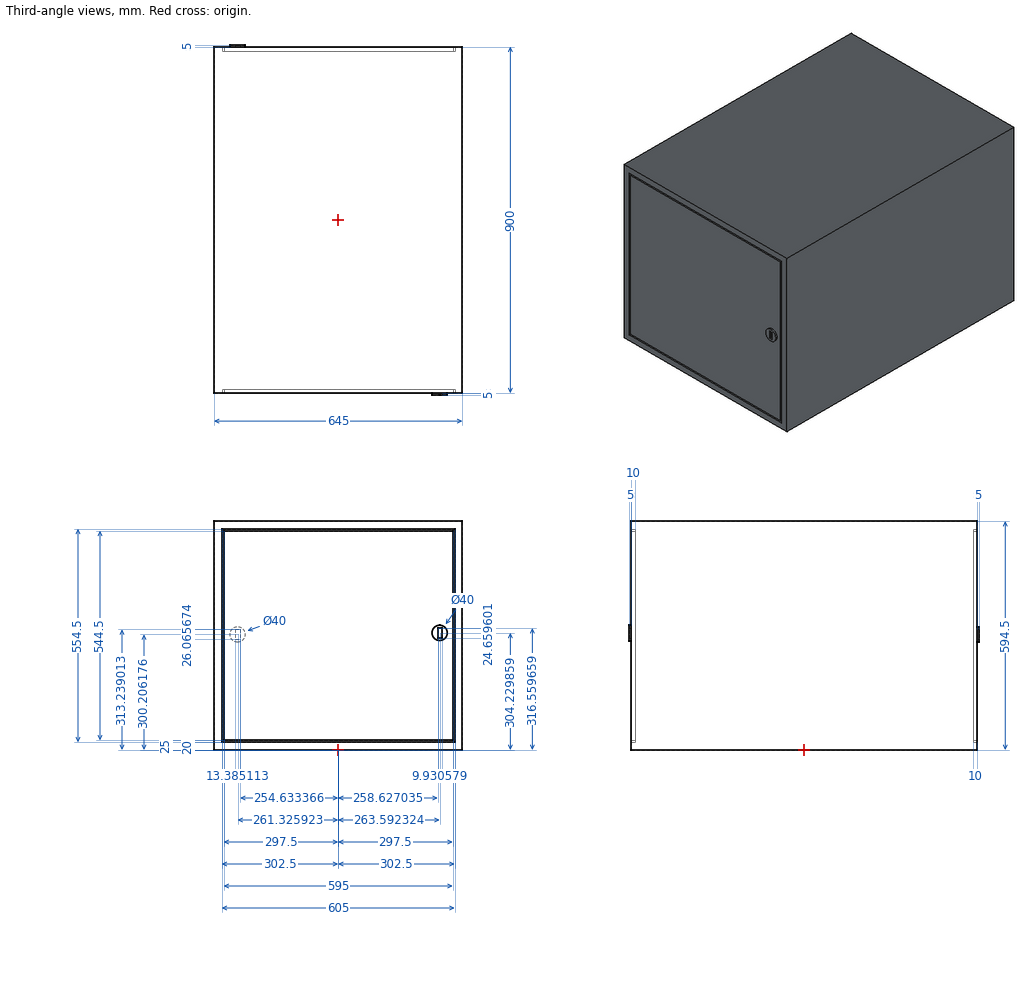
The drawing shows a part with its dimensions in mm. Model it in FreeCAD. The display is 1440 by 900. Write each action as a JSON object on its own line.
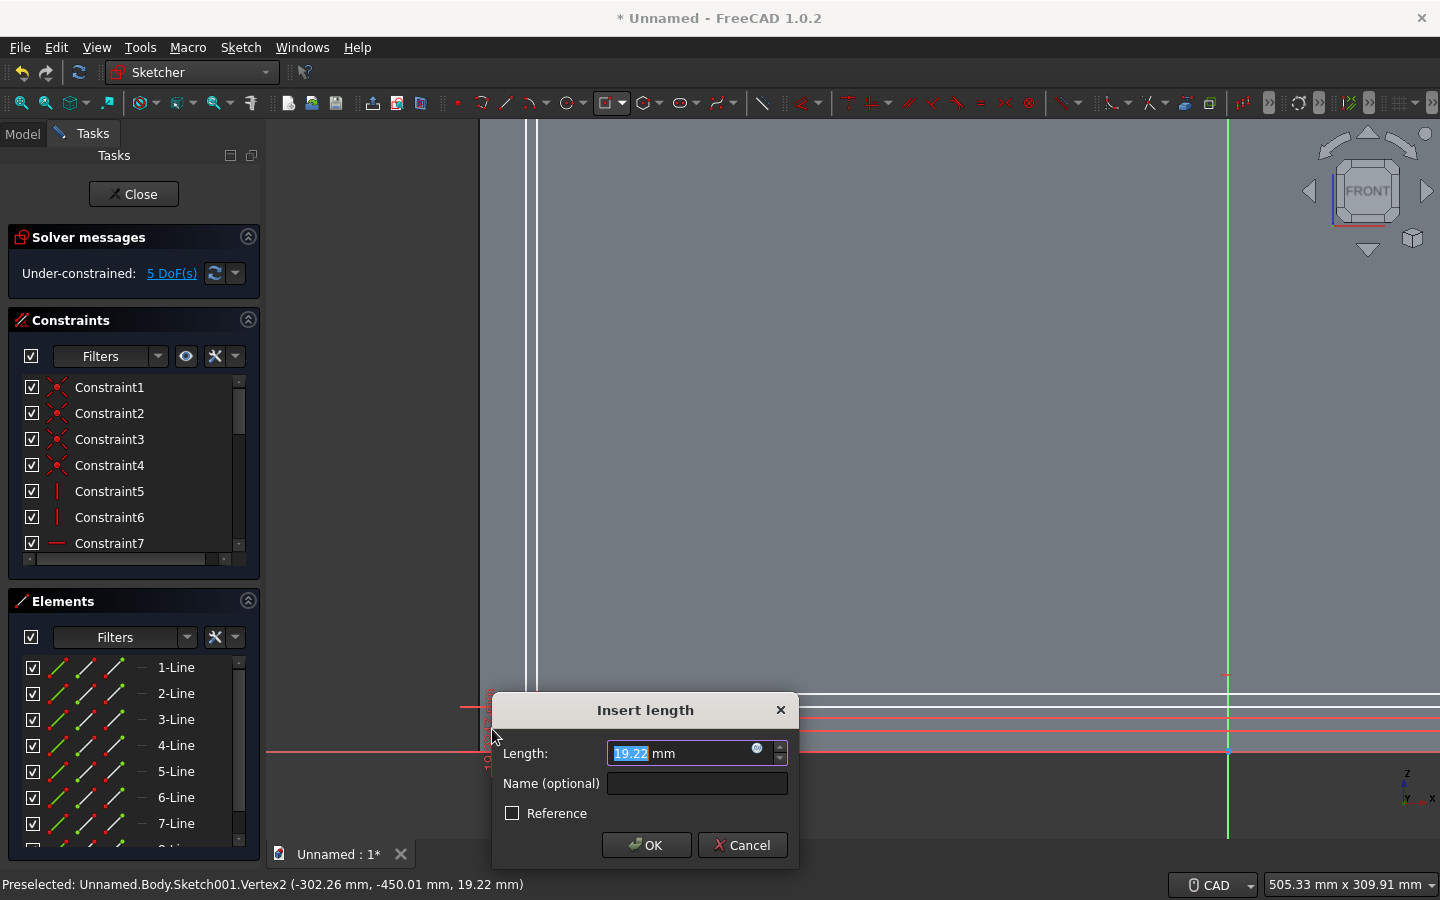
{"action": "type", "text": "20"}
{"action": "key", "text": "Return"}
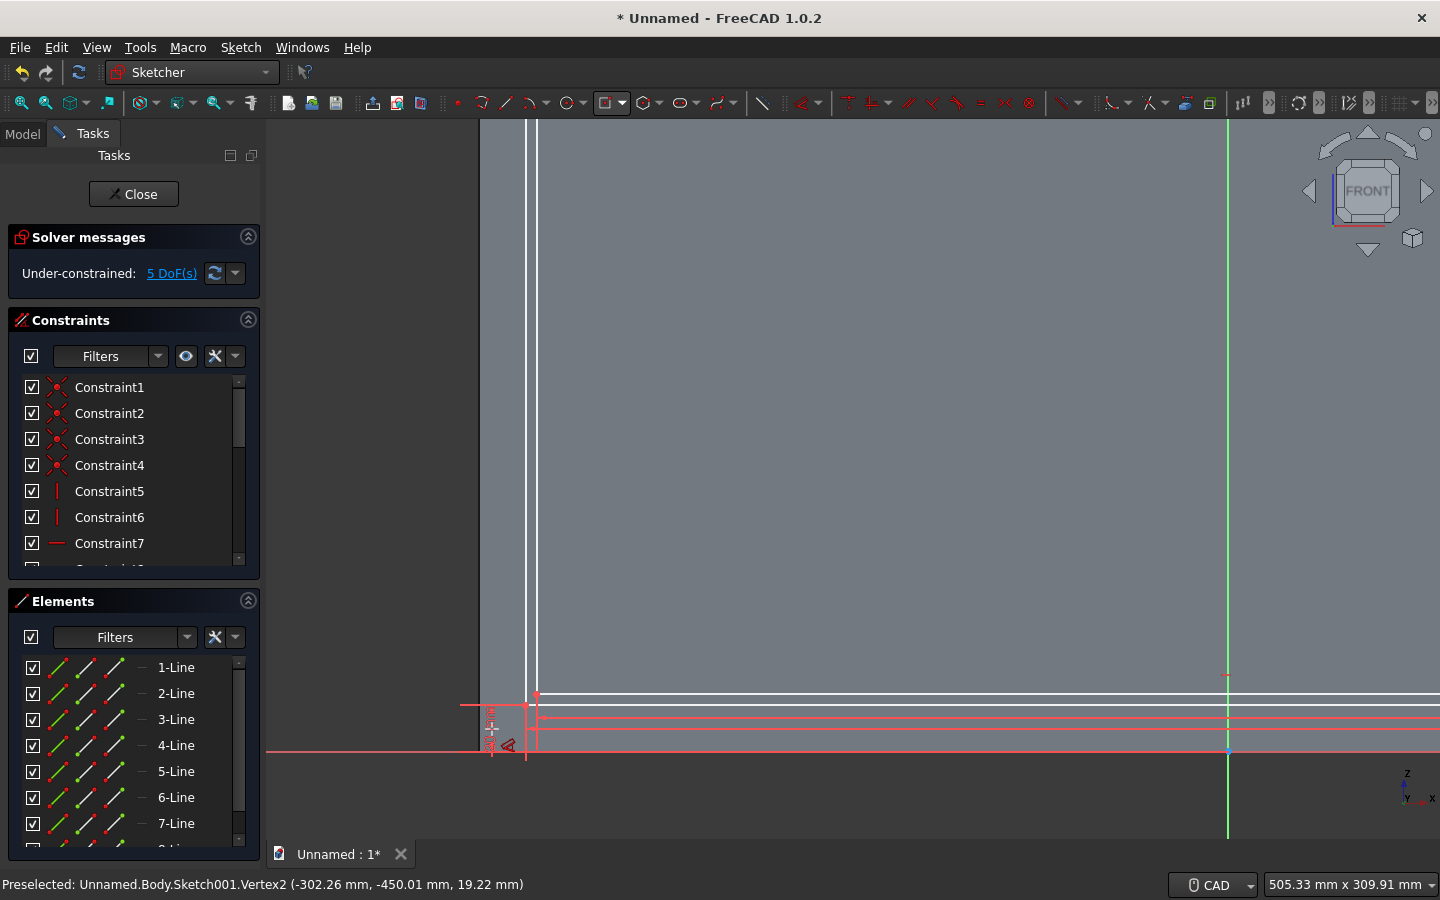
{"action": "left_click", "coordinate": [537, 694]}
{"action": "left_click", "coordinate": [503, 703]}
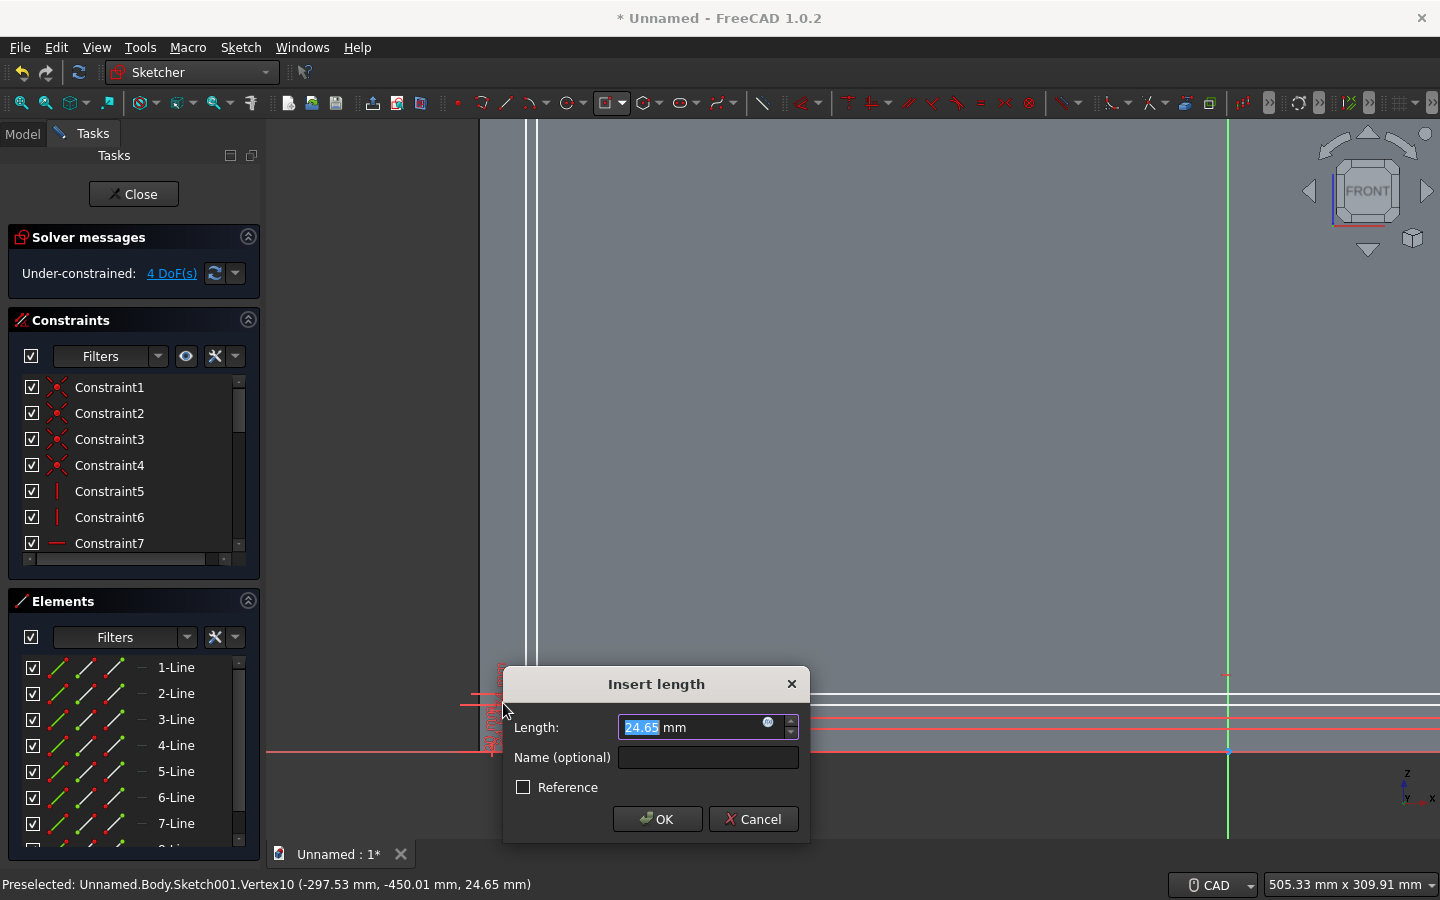
{"action": "type", "text": "25"}
{"action": "key", "text": "Return"}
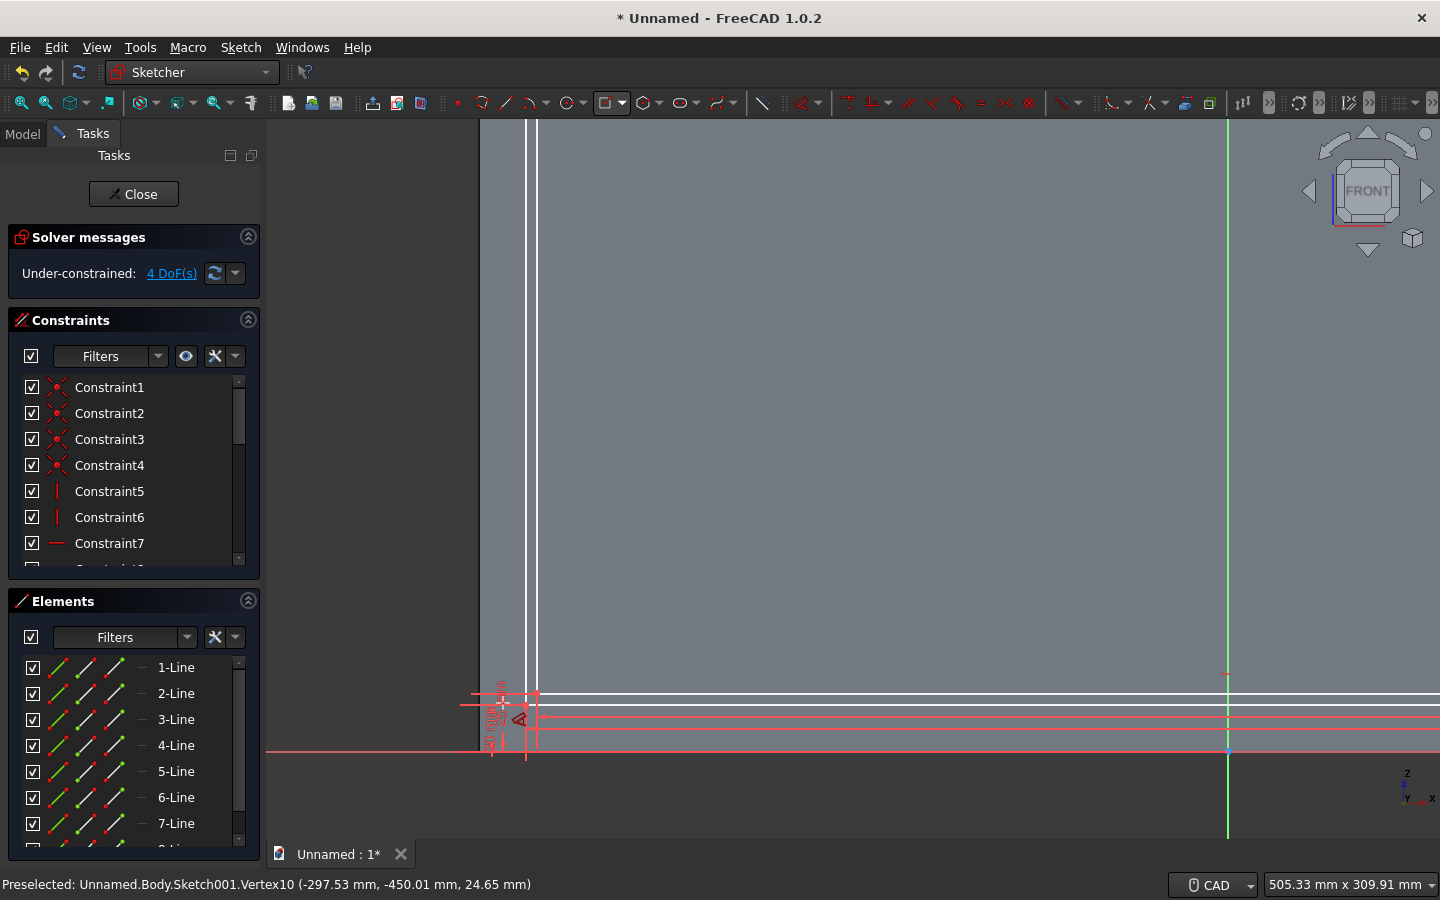
{"action": "scroll", "coordinate": [526, 319], "scroll_direction": "up", "scroll_amount": 2}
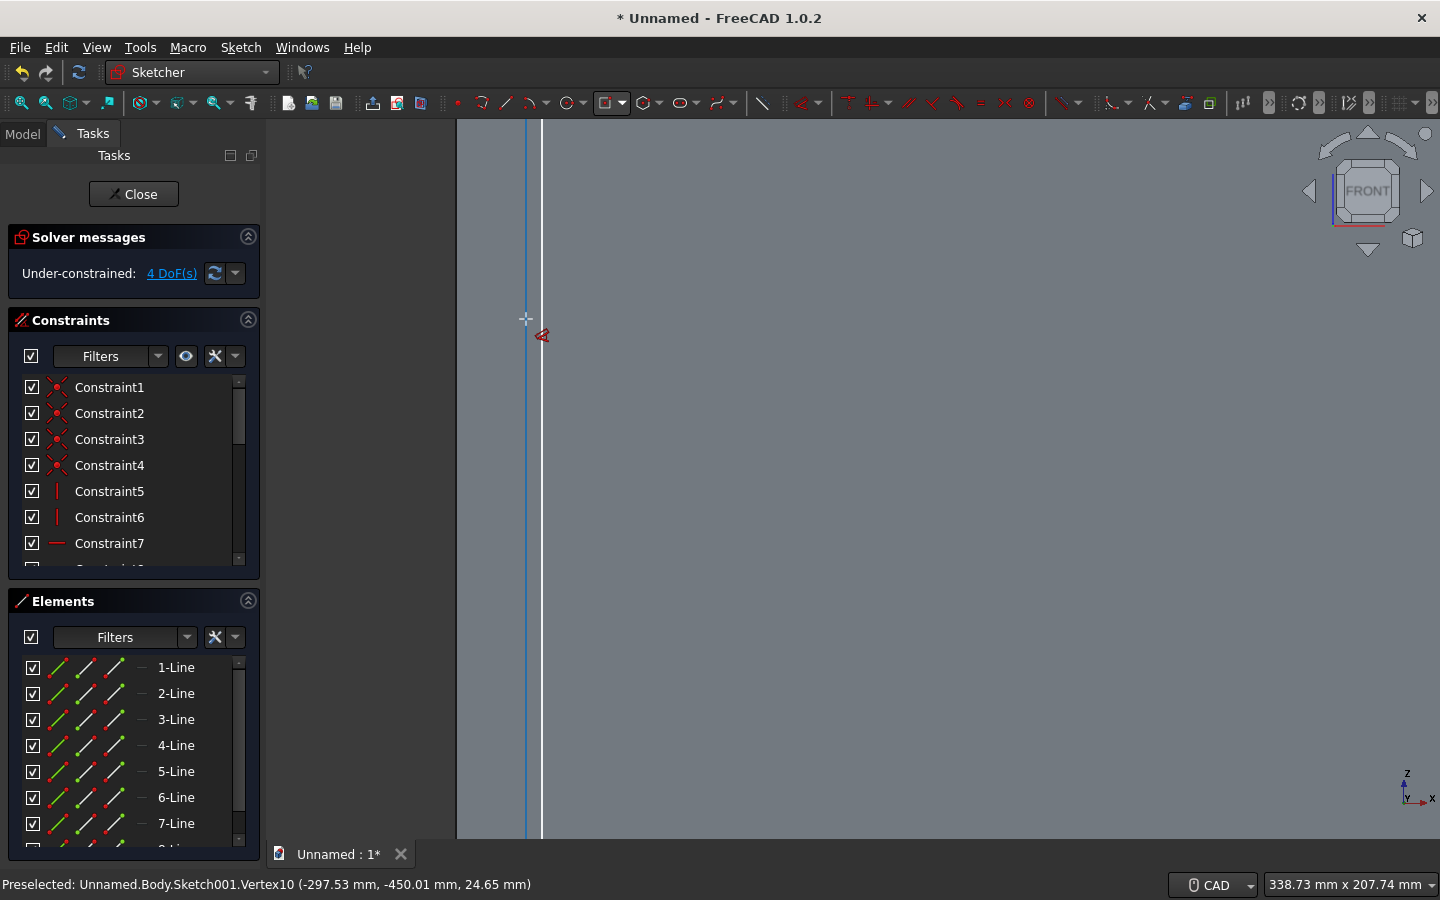
{"action": "left_click", "coordinate": [526, 319]}
{"action": "left_click", "coordinate": [492, 479]}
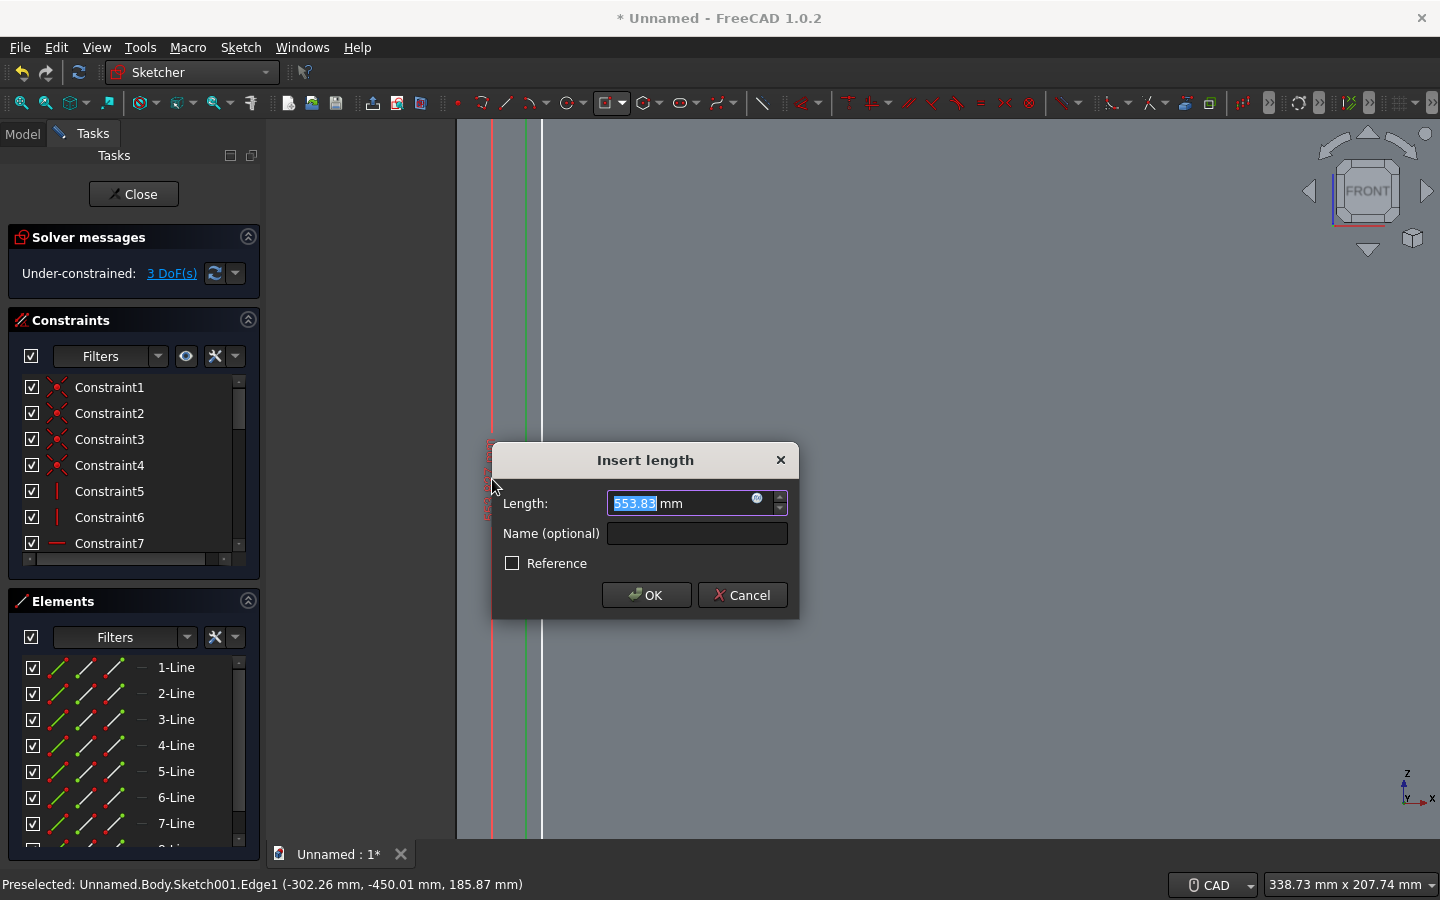
{"action": "type", "text": "554.5"}
{"action": "key", "text": "Return"}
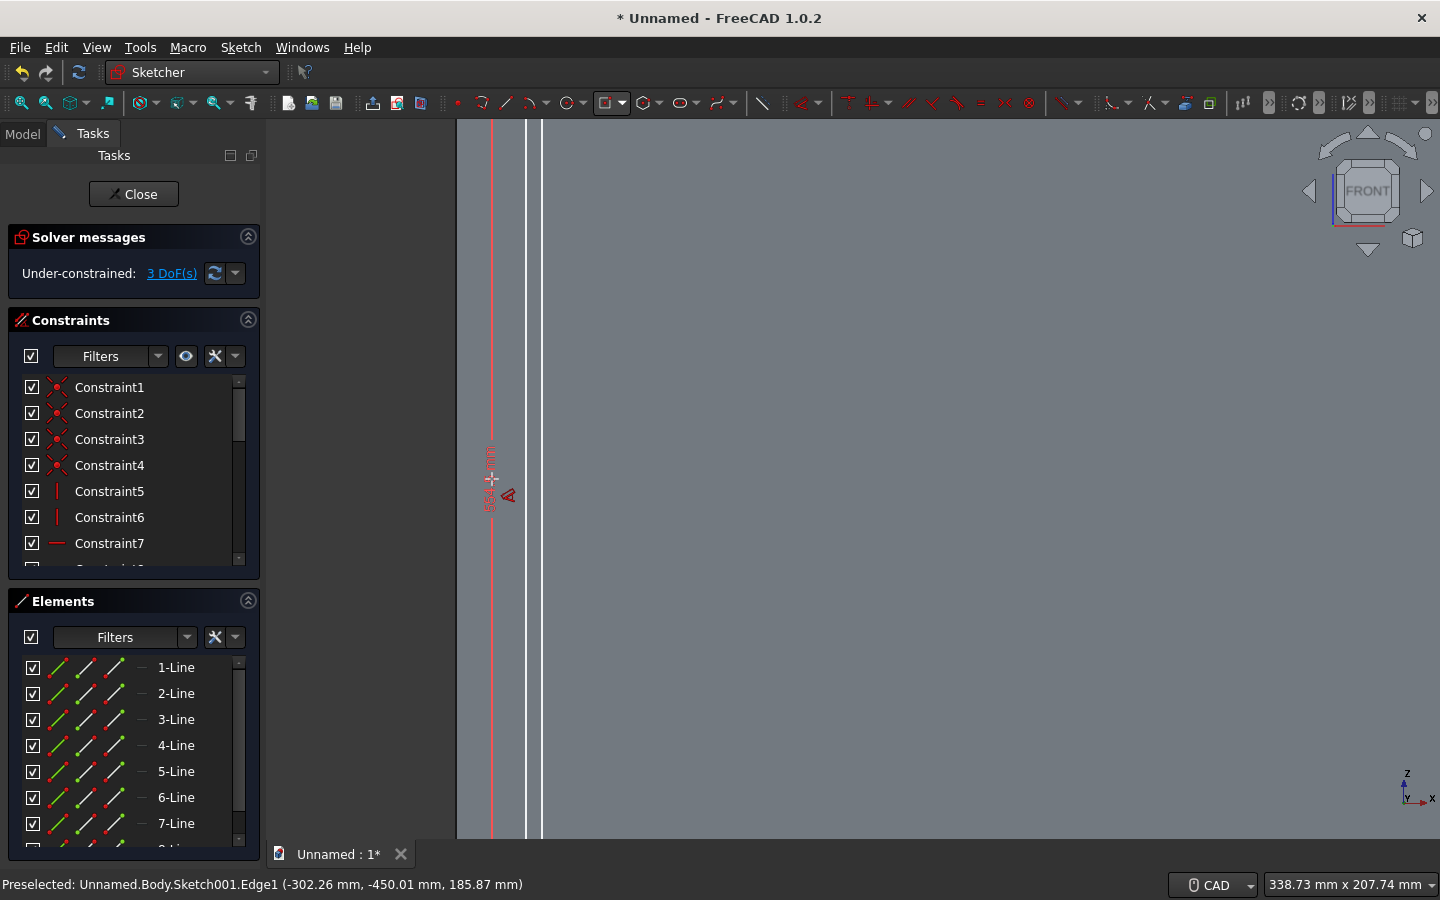
{"action": "left_click", "coordinate": [542, 312]}
{"action": "left_click", "coordinate": [508, 326]}